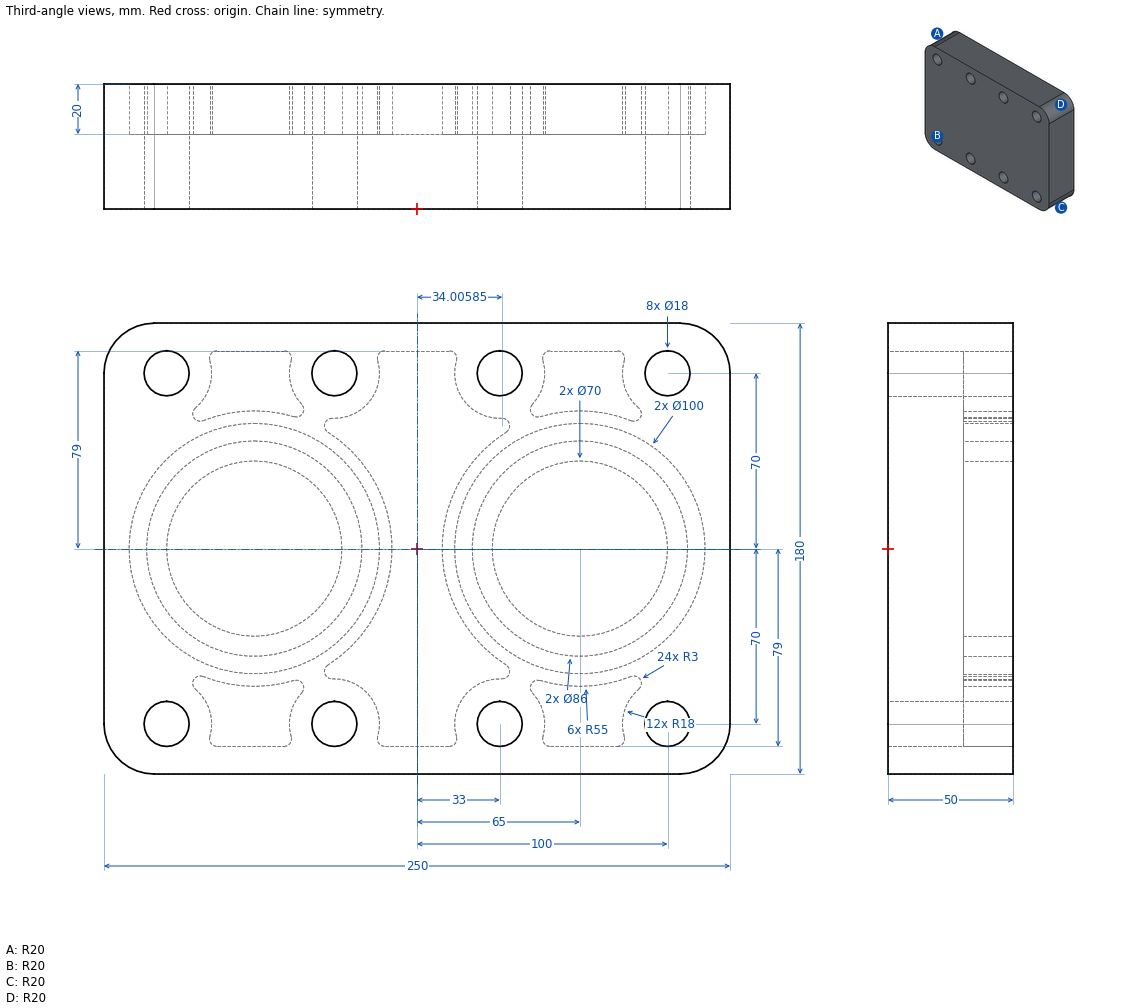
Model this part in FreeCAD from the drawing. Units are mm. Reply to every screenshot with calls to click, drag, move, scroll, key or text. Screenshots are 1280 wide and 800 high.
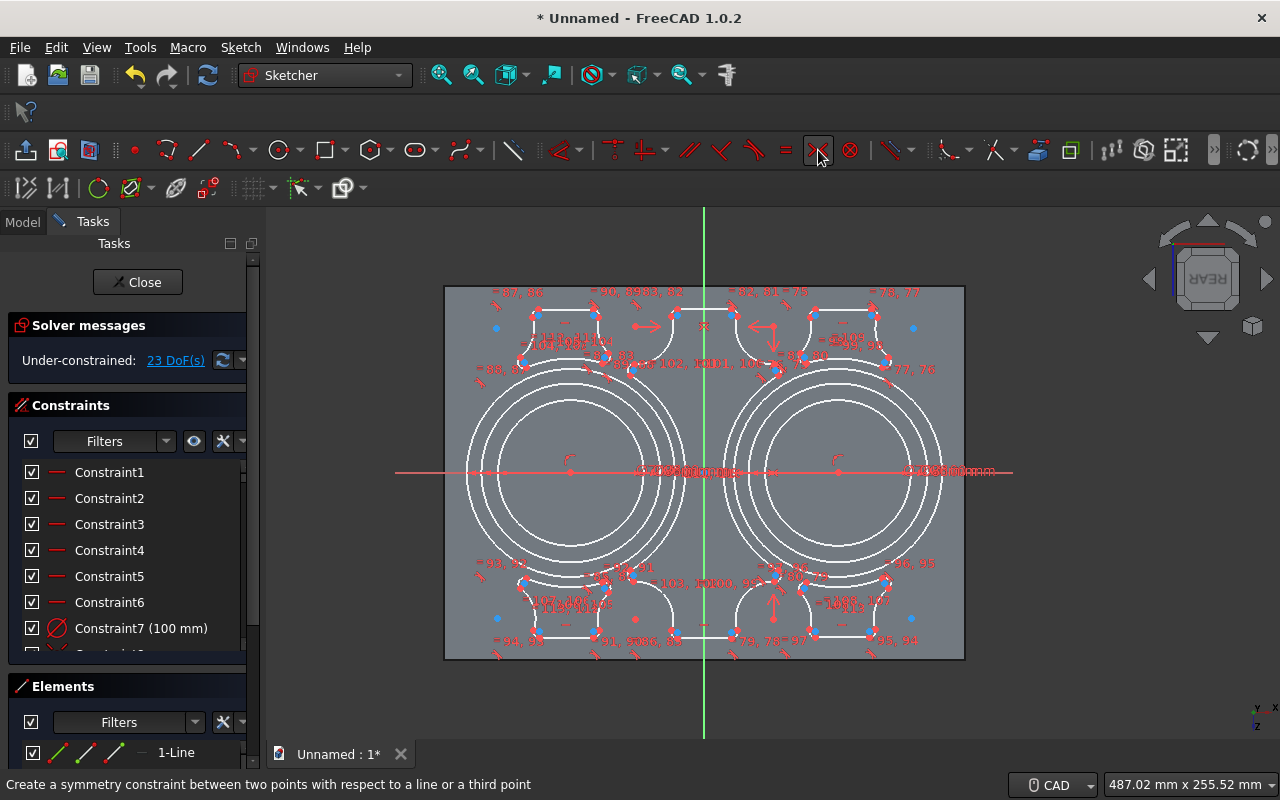
scroll(775, 576, up, 4)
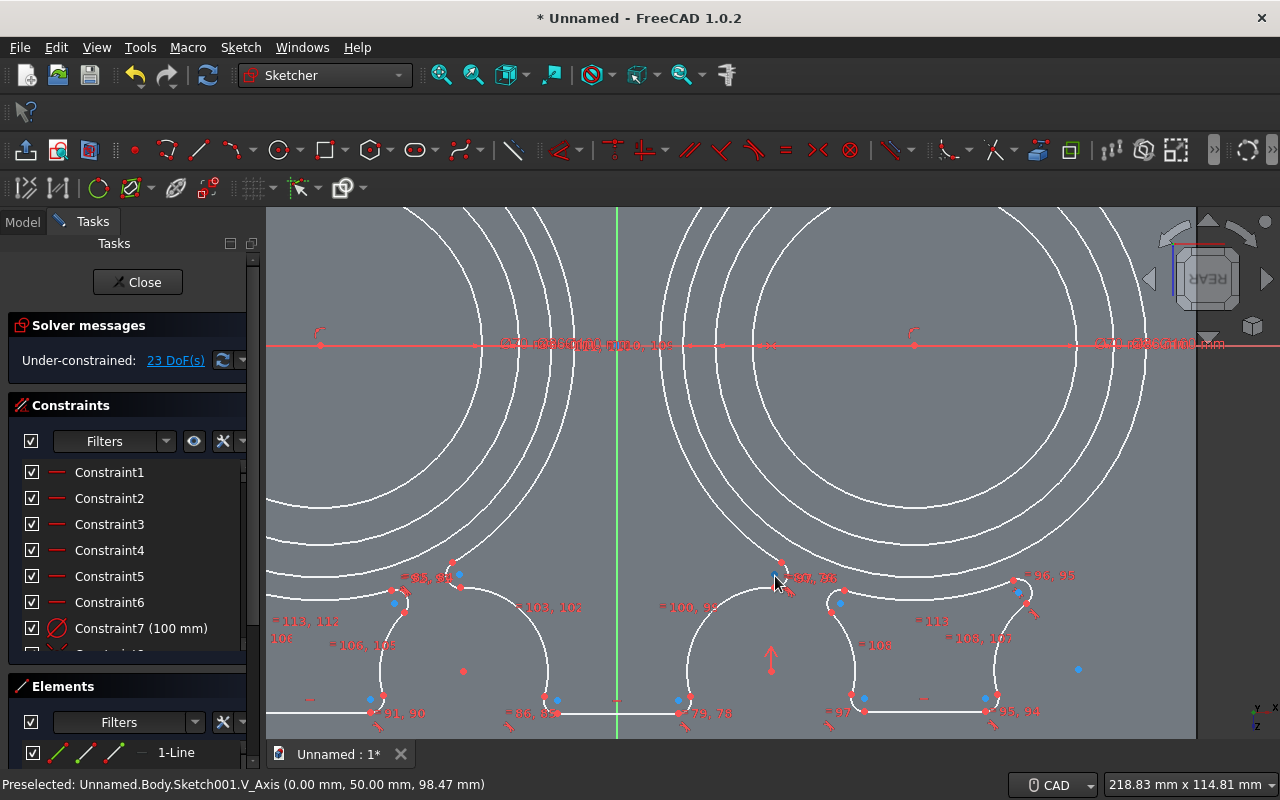
click(774, 574)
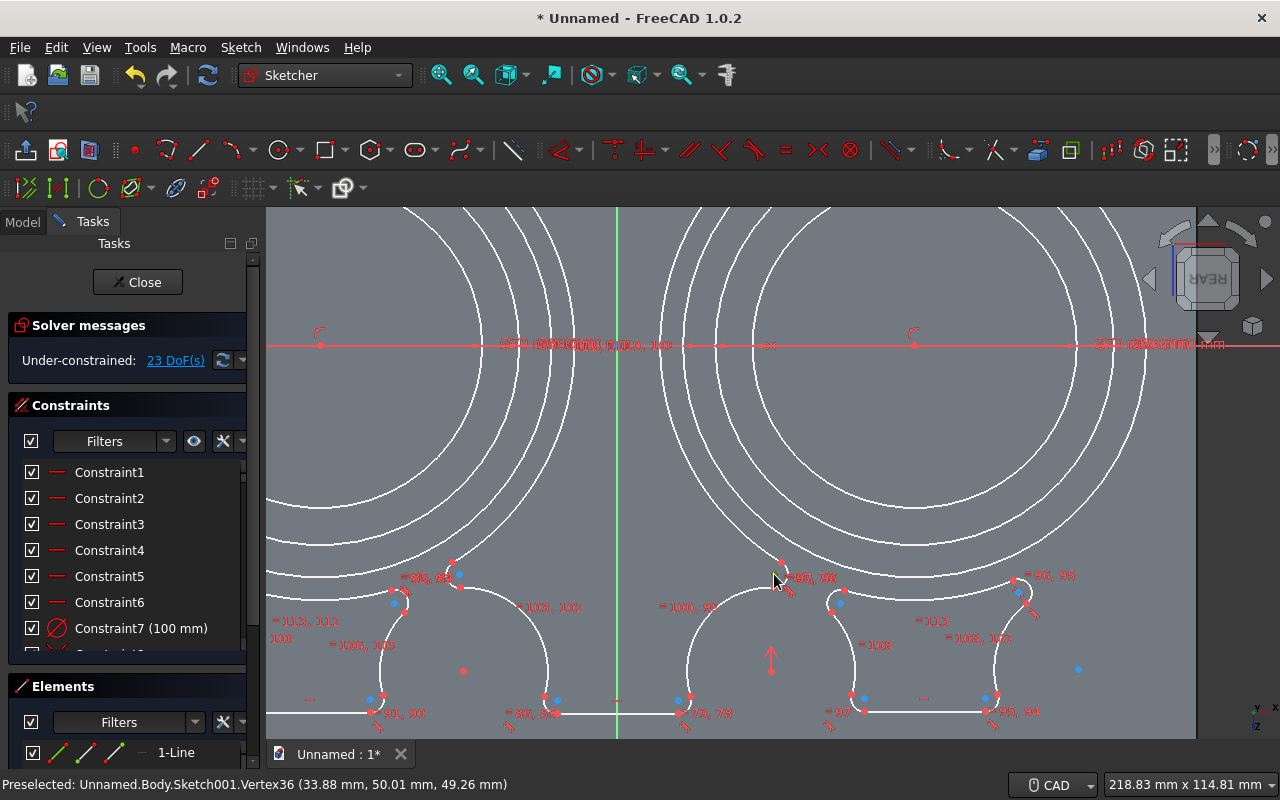
click(460, 574)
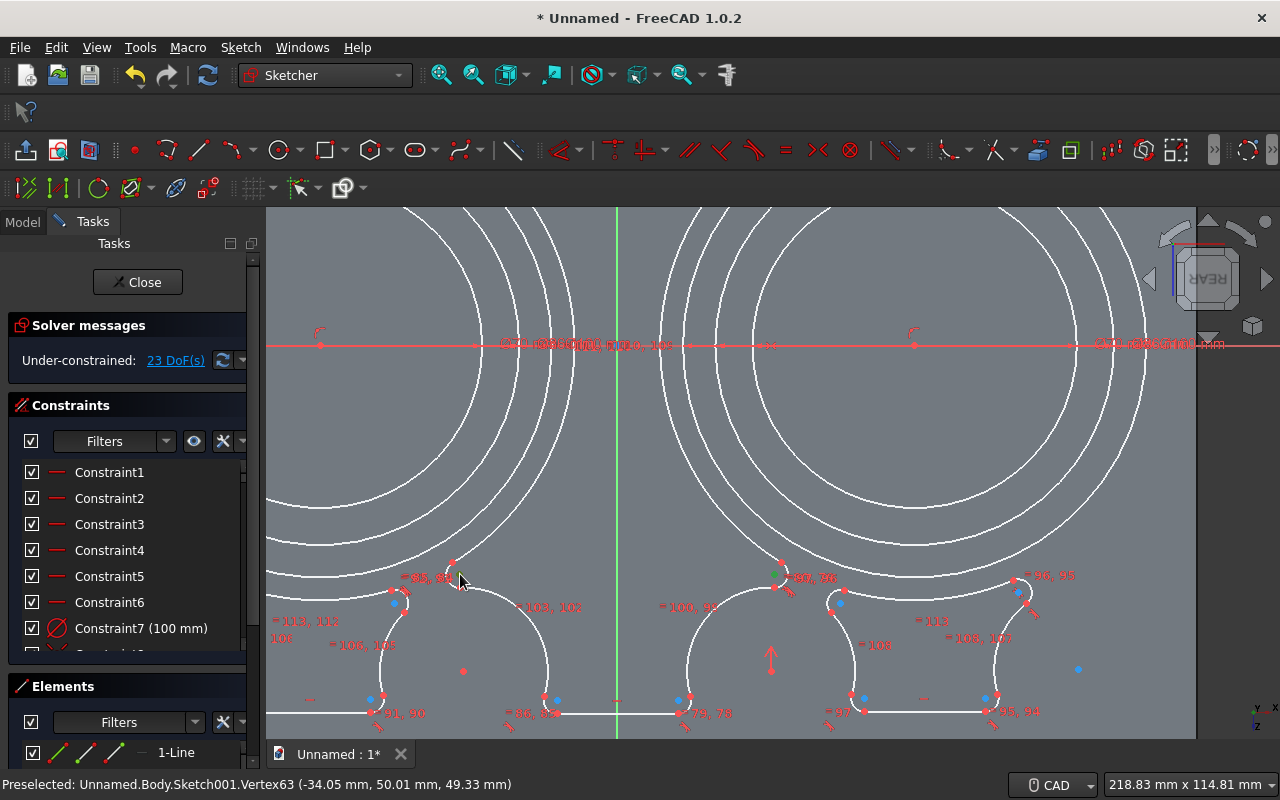
click(617, 677)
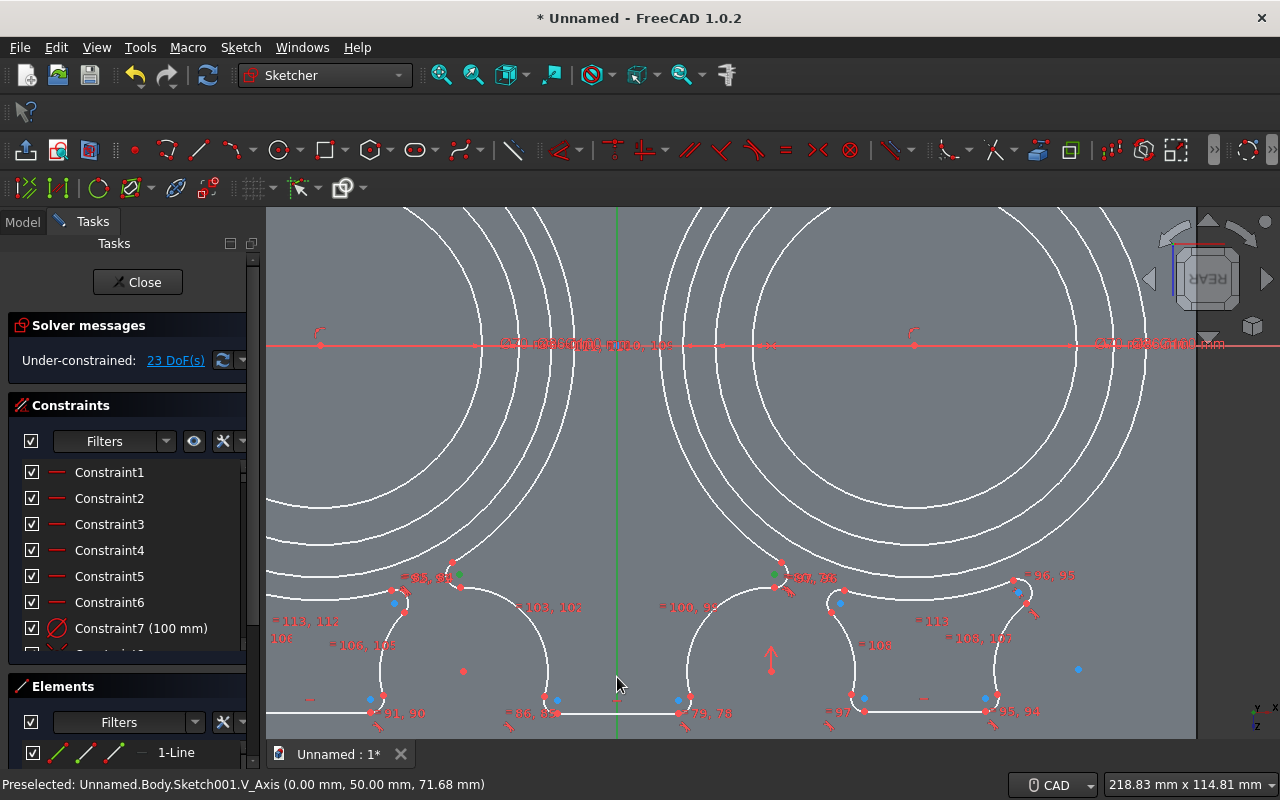
click(818, 150)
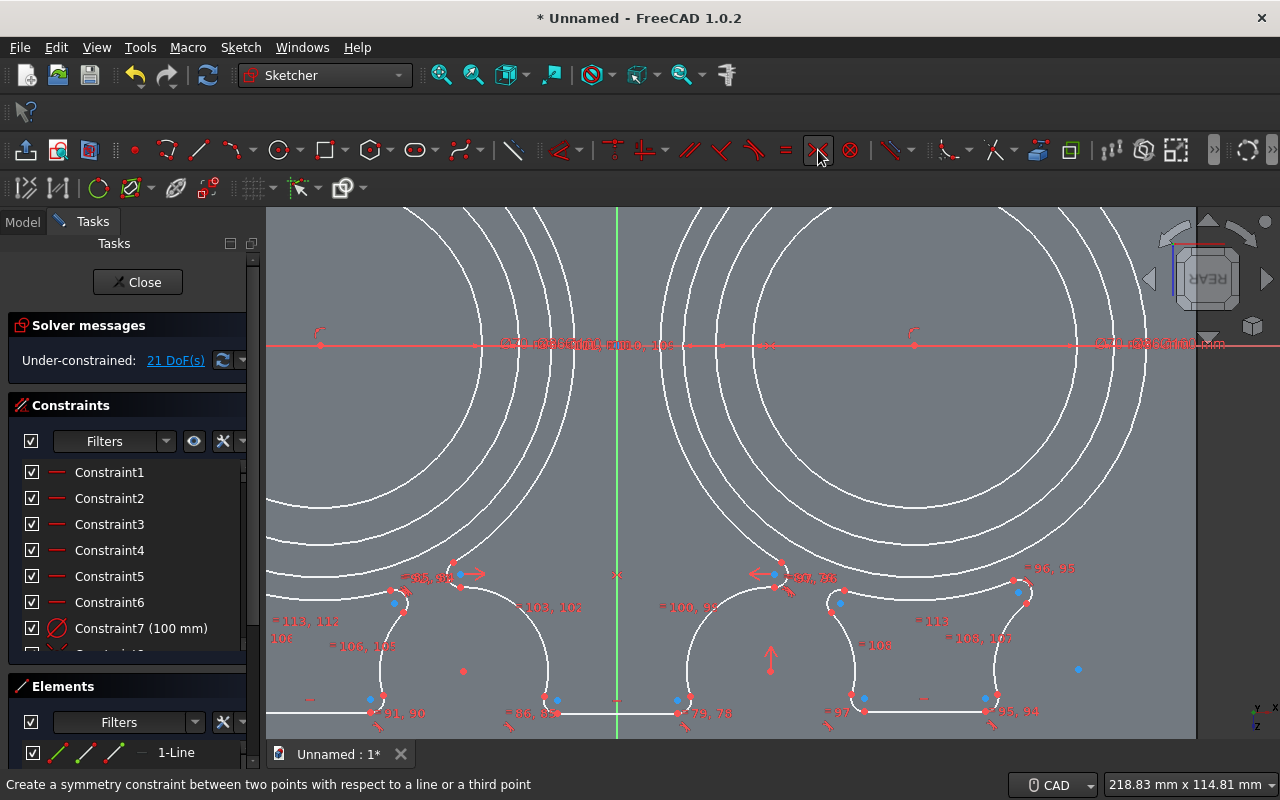
scroll(776, 577, down, 4)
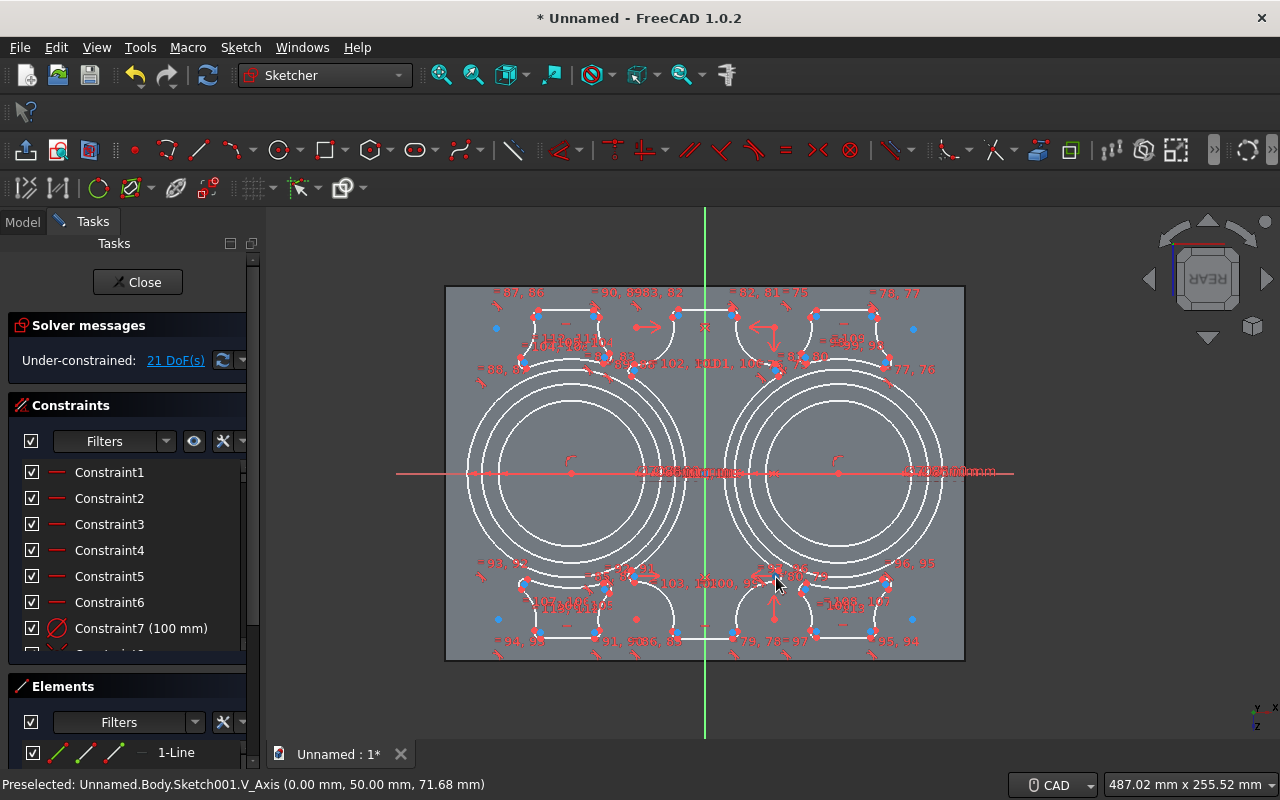
scroll(678, 316, up, 4)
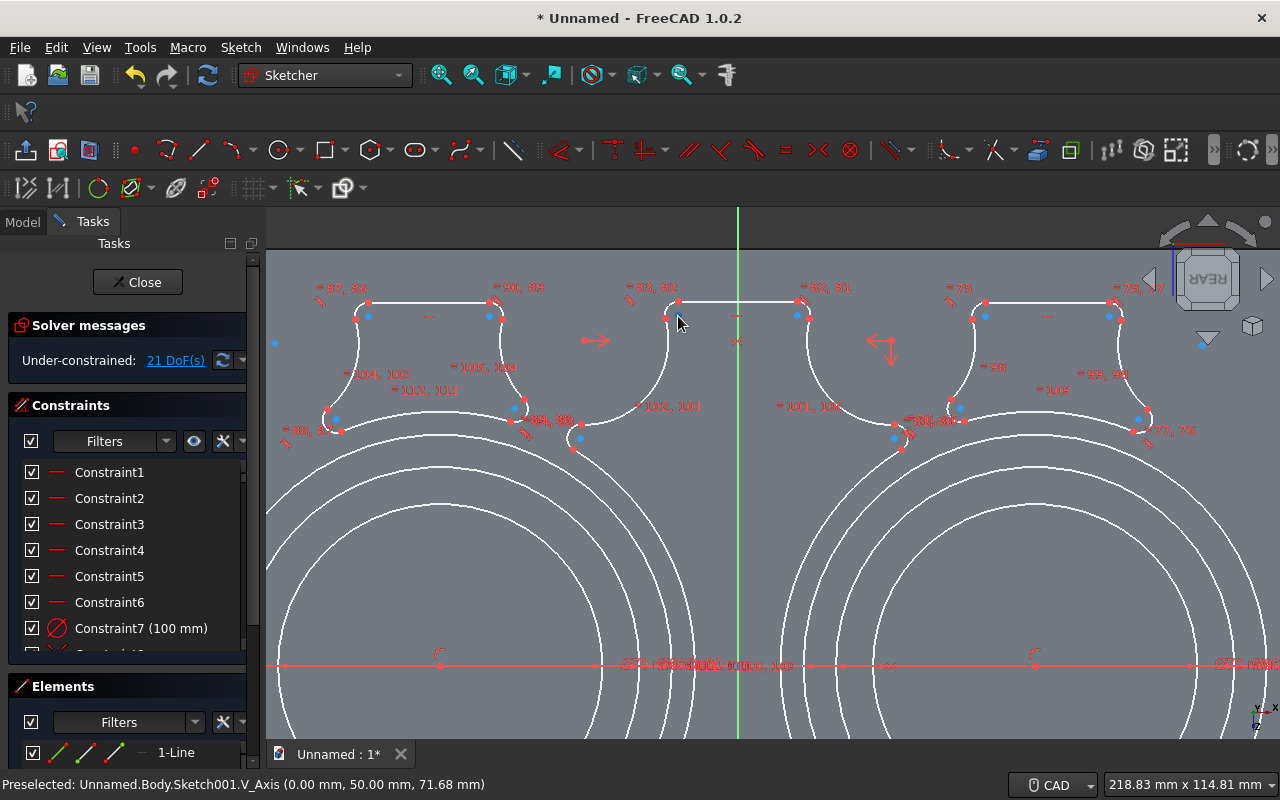
click(678, 315)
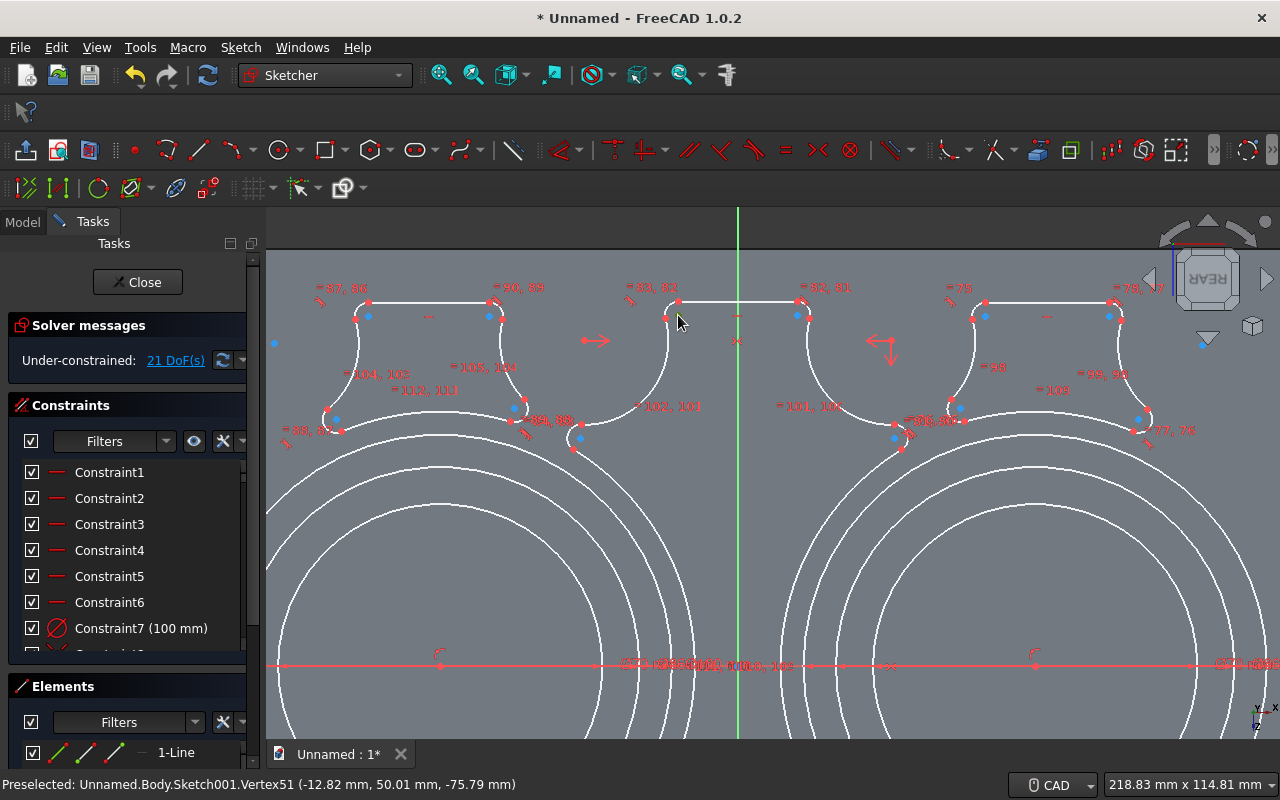
scroll(677, 315, down, 4)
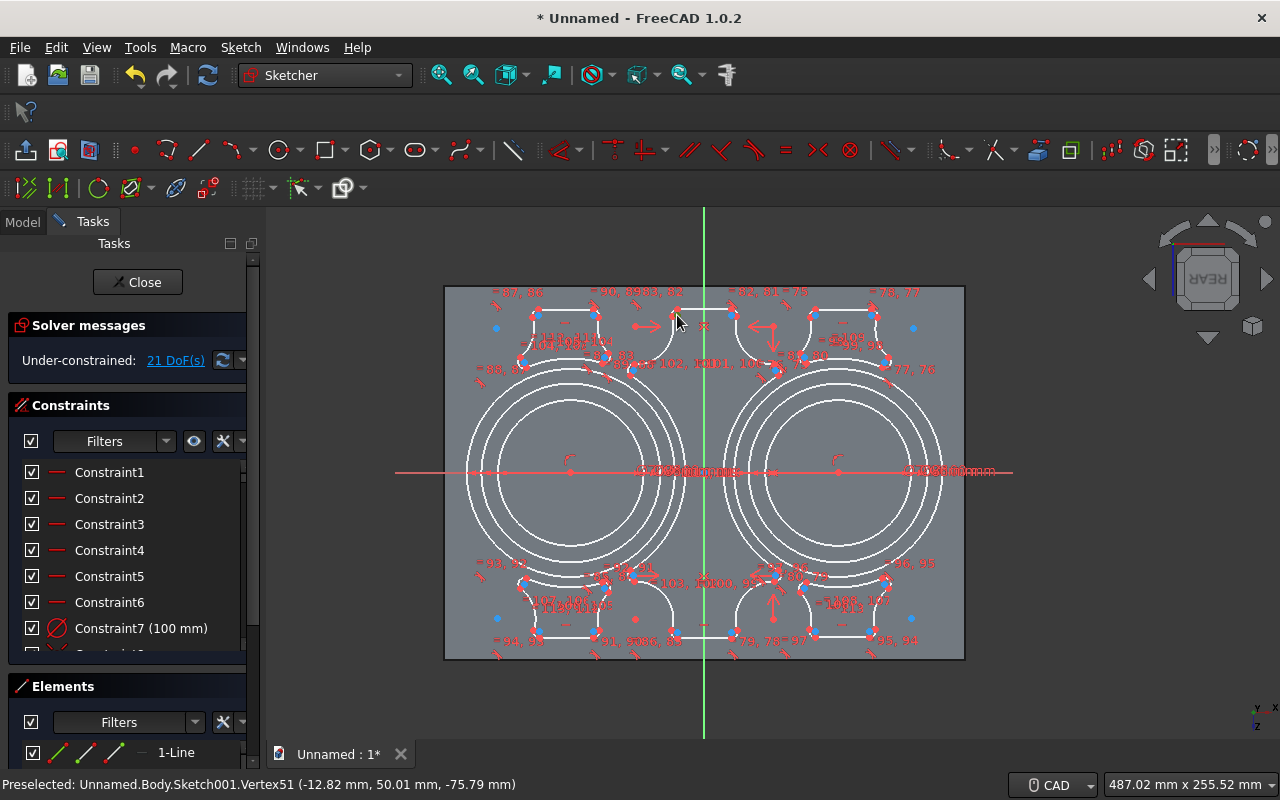
scroll(677, 632, up, 4)